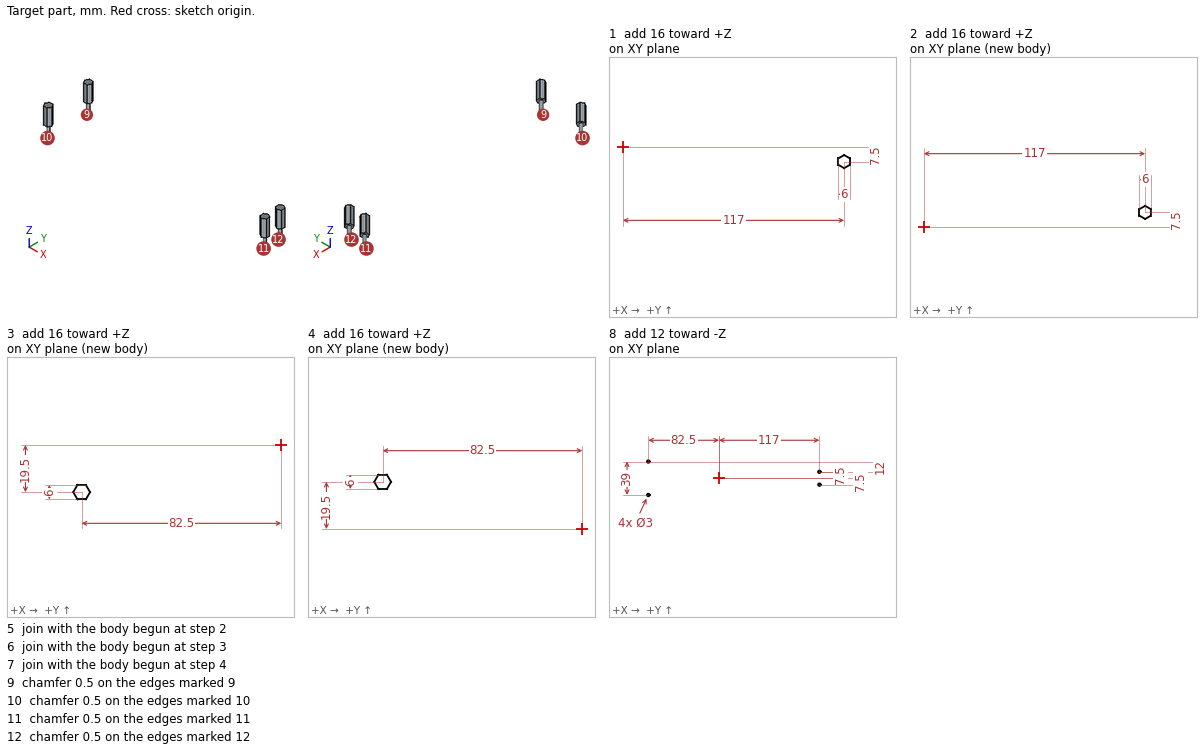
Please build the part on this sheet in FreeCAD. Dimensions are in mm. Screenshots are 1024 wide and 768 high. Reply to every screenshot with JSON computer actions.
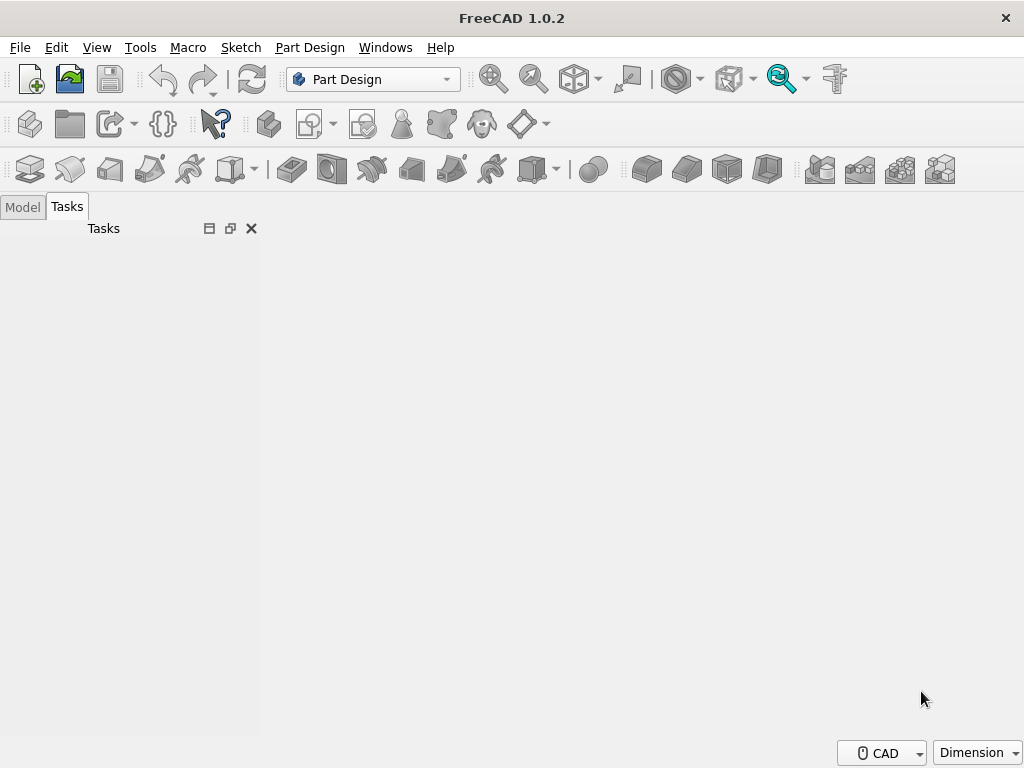
{"action": "left_click", "coordinate": [30, 80]}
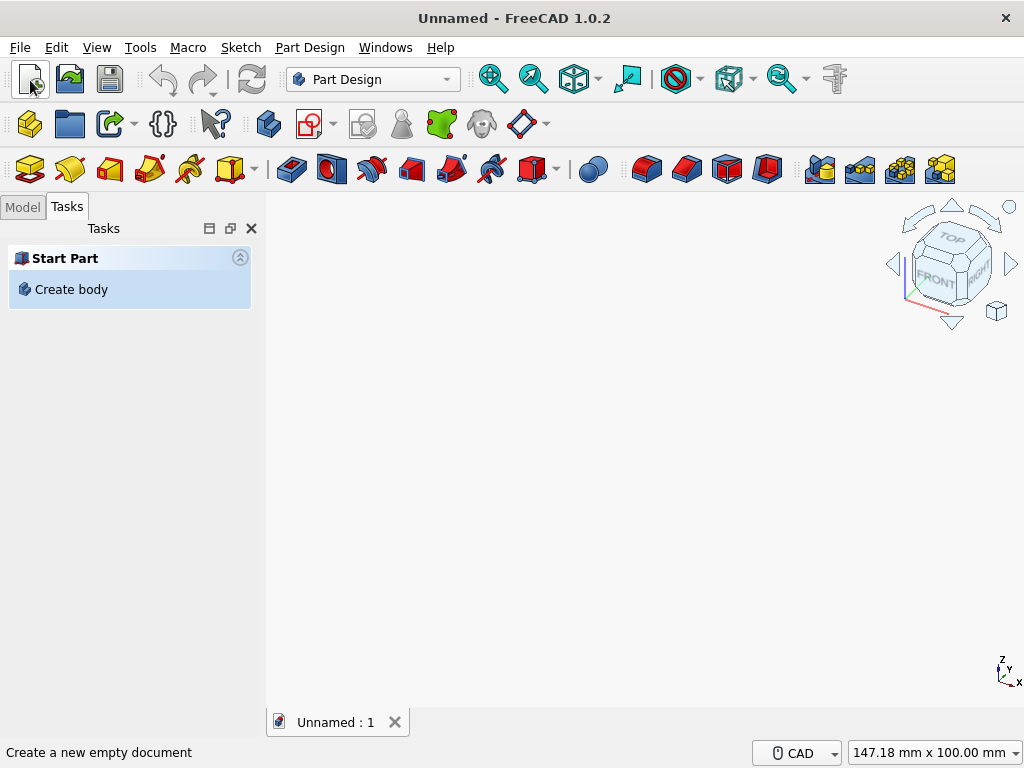
{"action": "left_click", "coordinate": [310, 124]}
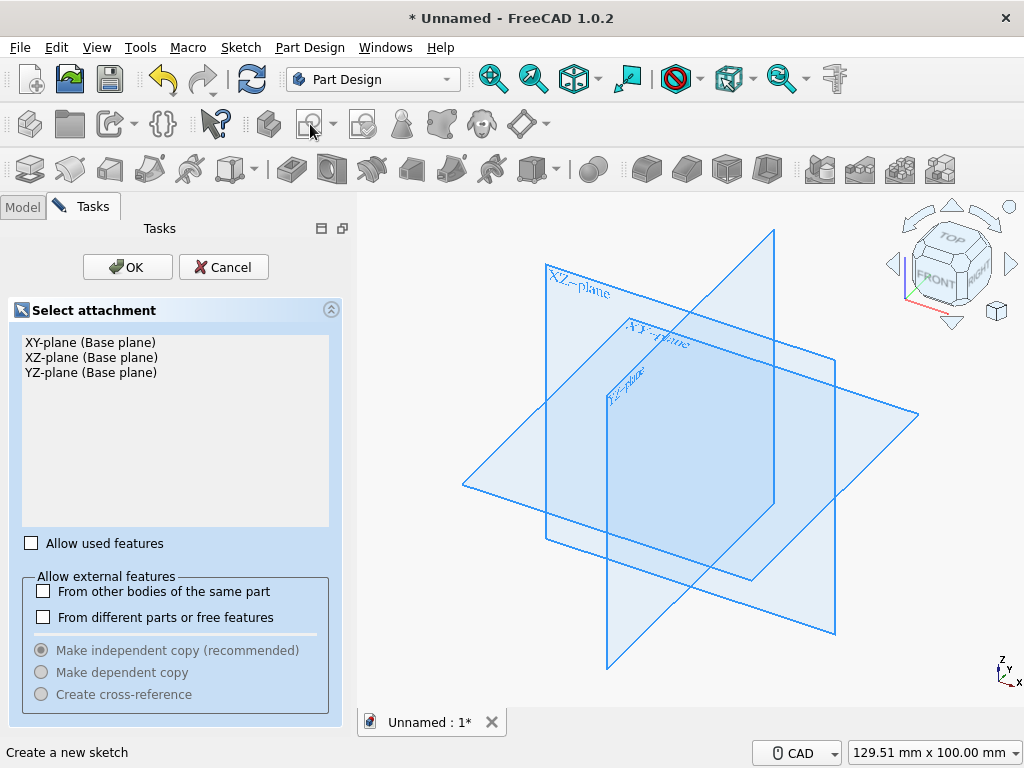
{"action": "left_click", "coordinate": [82, 342]}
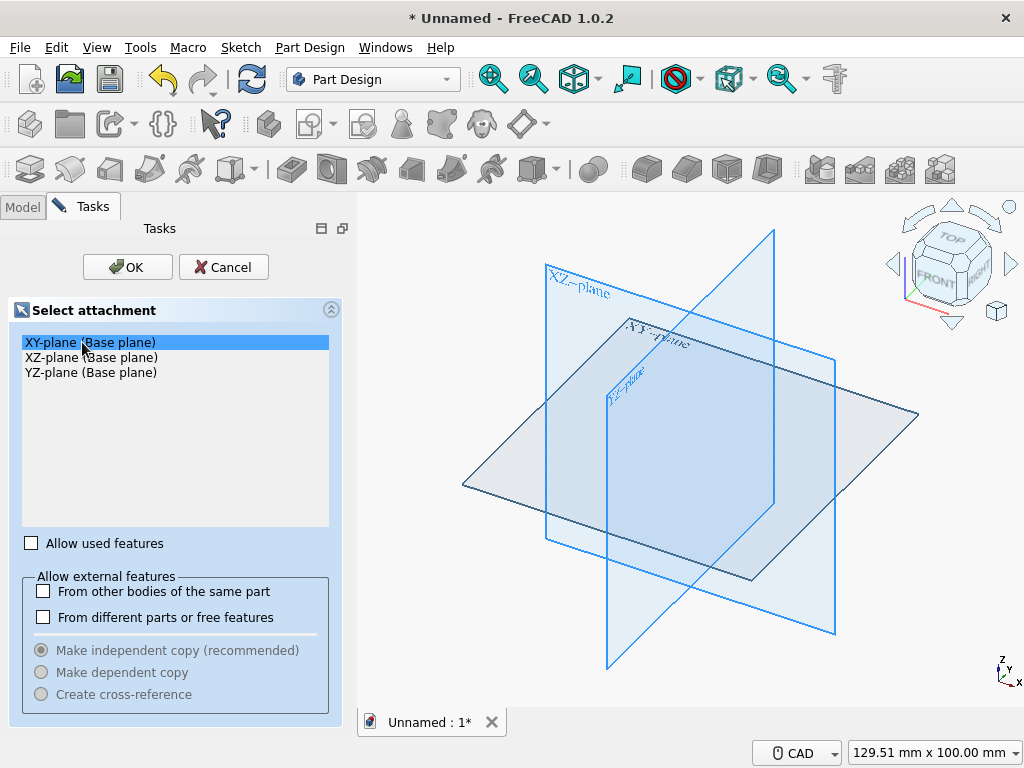
{"action": "left_click", "coordinate": [128, 267]}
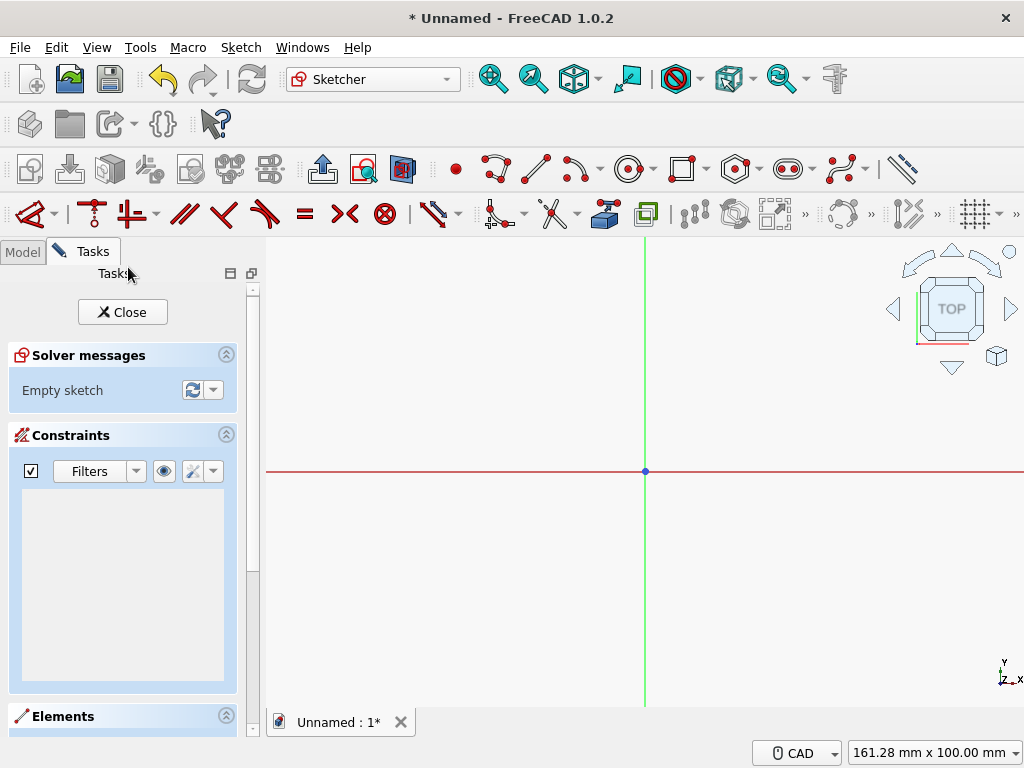
{"action": "scroll", "coordinate": [576, 472], "scroll_direction": "down", "scroll_amount": 5}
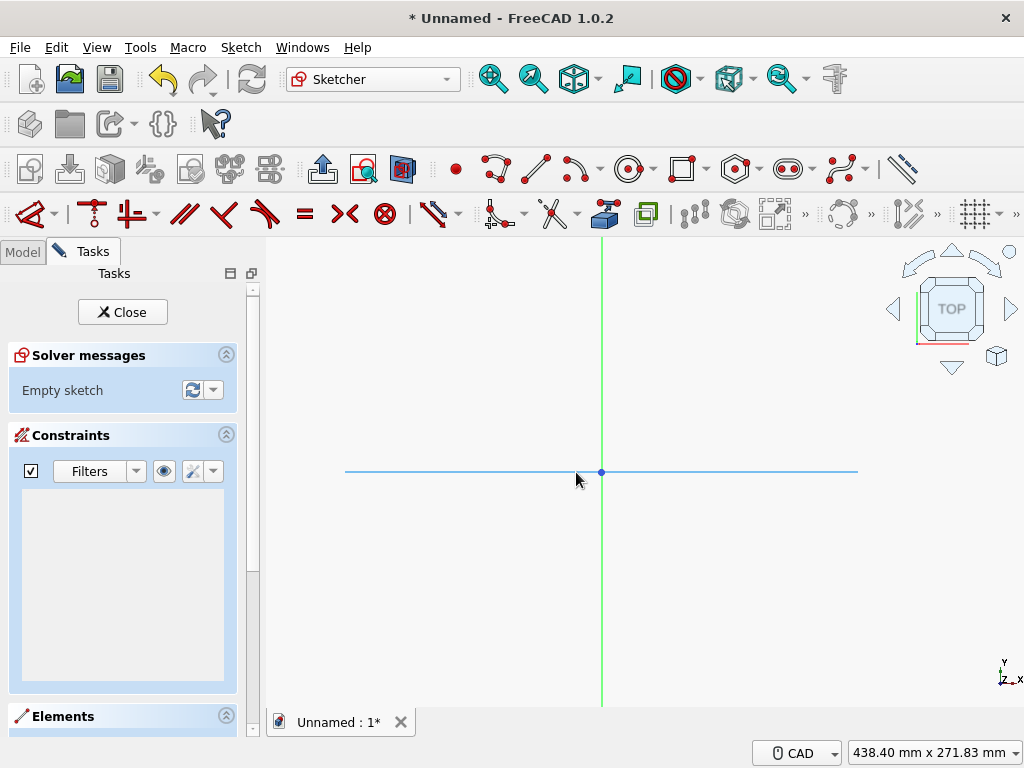
{"action": "scroll", "coordinate": [816, 486], "scroll_direction": "up", "scroll_amount": 15}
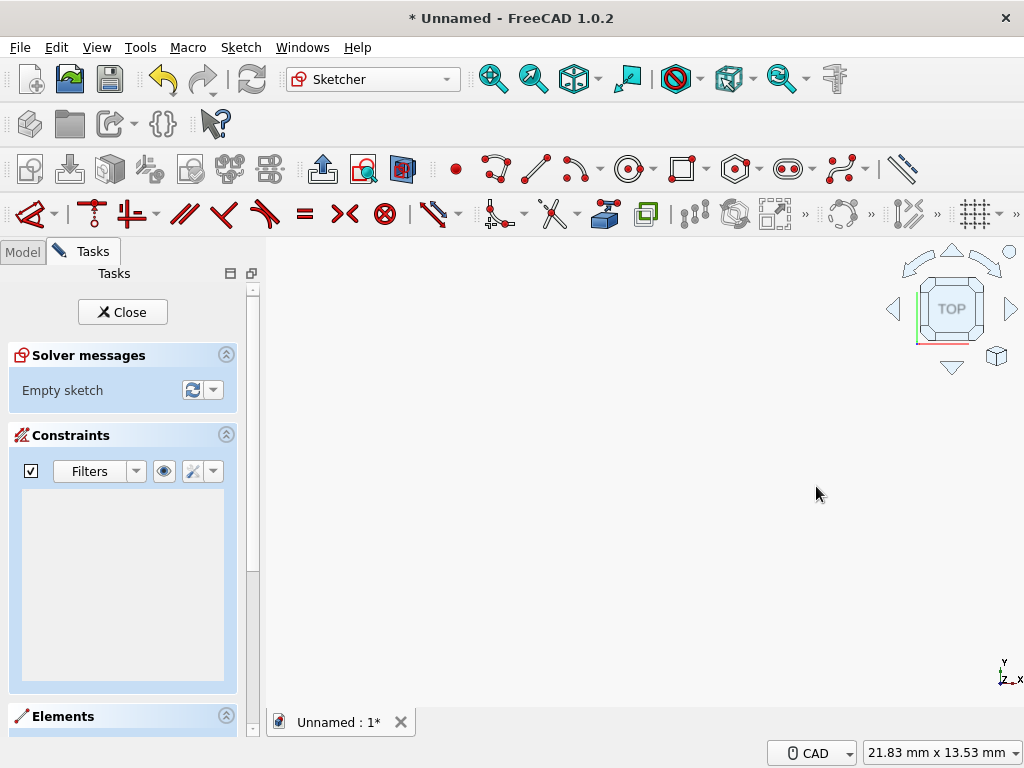
{"action": "left_click", "coordinate": [736, 170]}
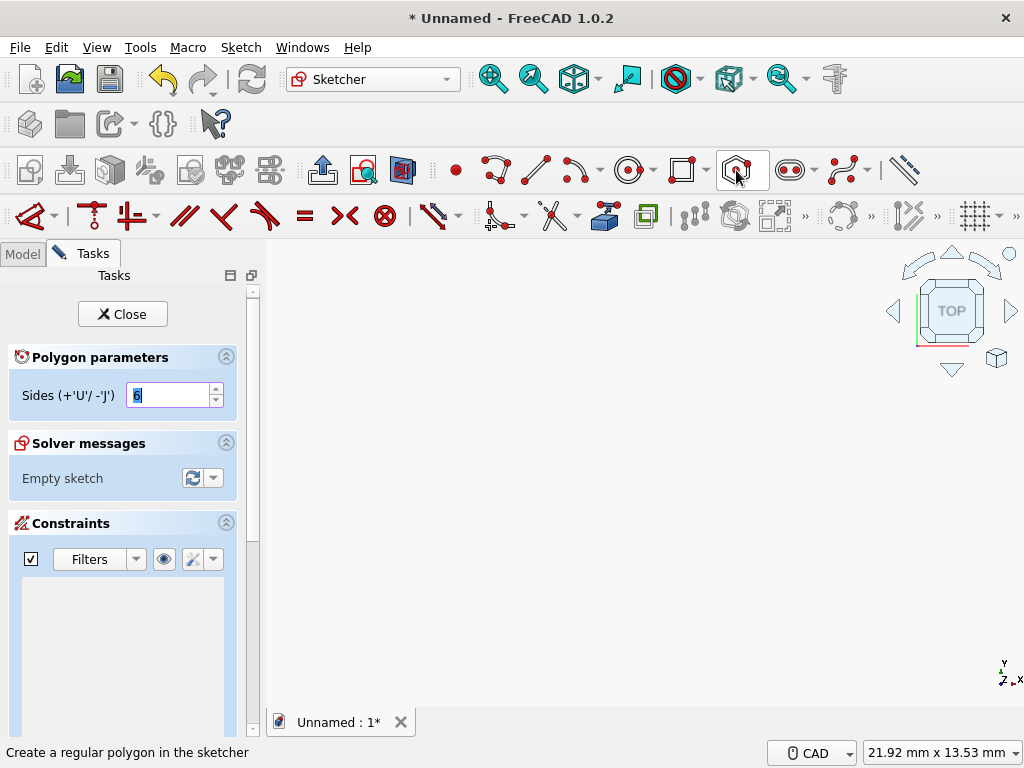
{"action": "left_click", "coordinate": [560, 463]}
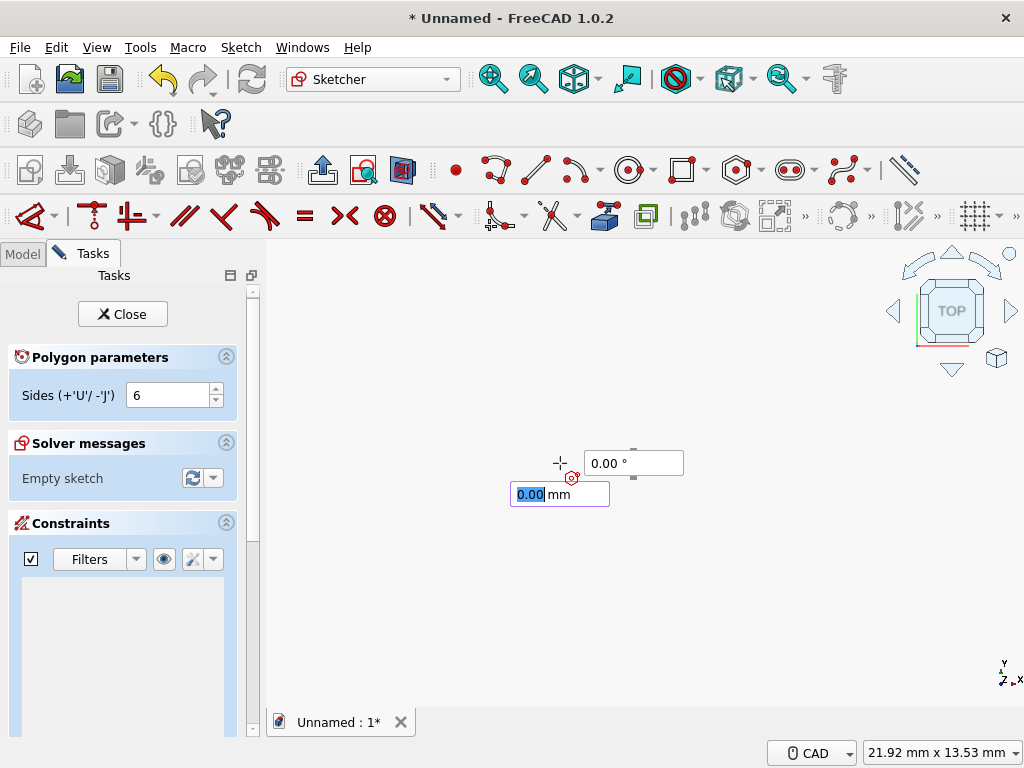
{"action": "left_click", "coordinate": [560, 582]}
{"action": "right_click", "coordinate": [560, 582]}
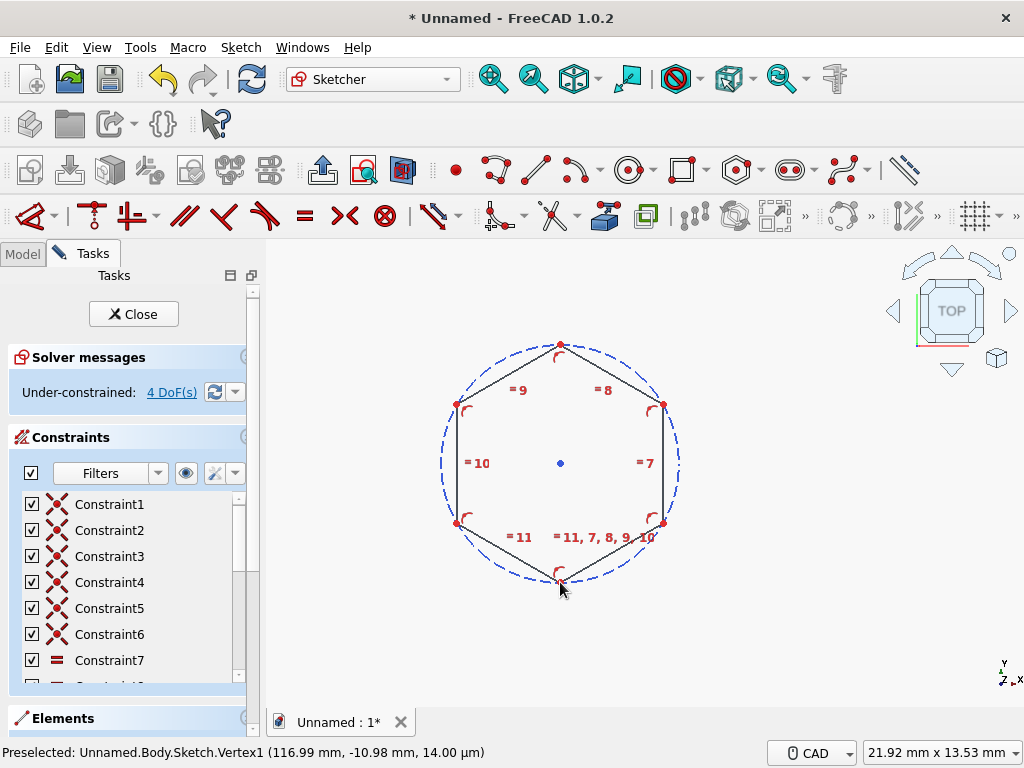
{"action": "left_click", "coordinate": [663, 488]}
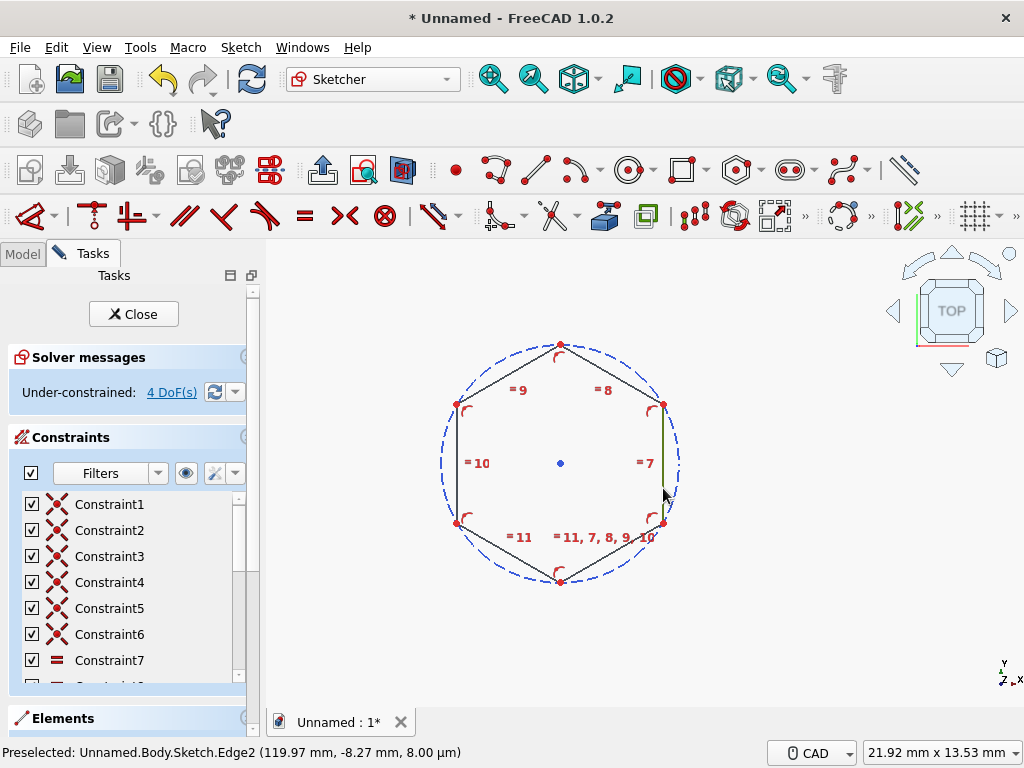
{"action": "left_click", "coordinate": [158, 216]}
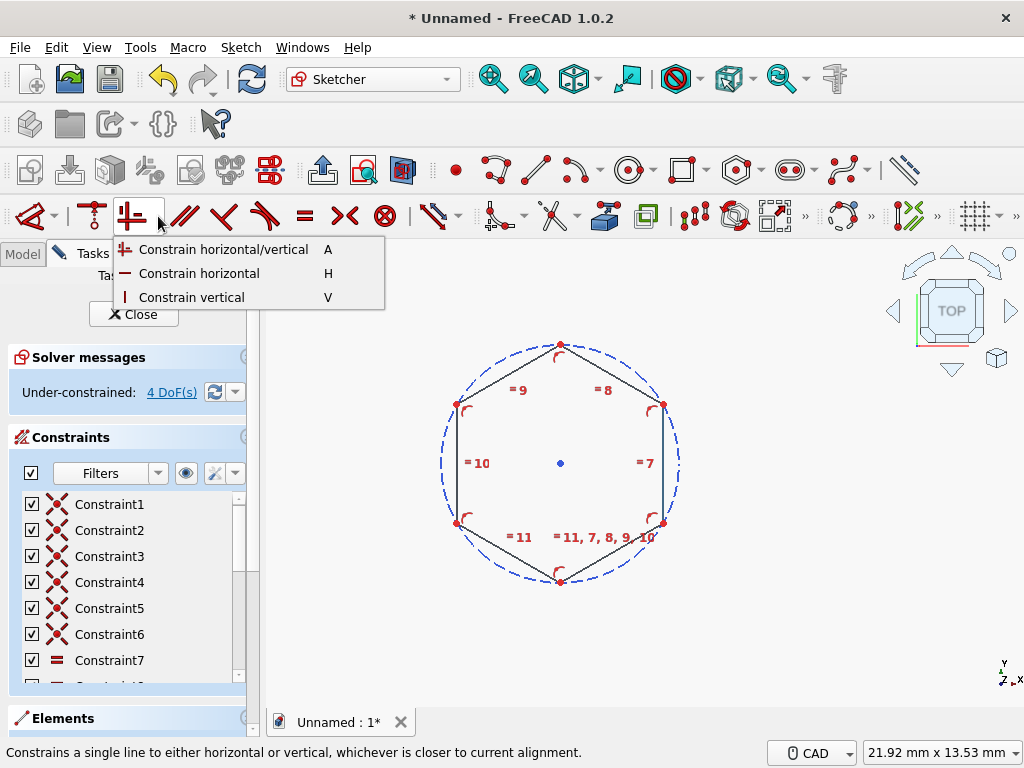
{"action": "left_click", "coordinate": [249, 297]}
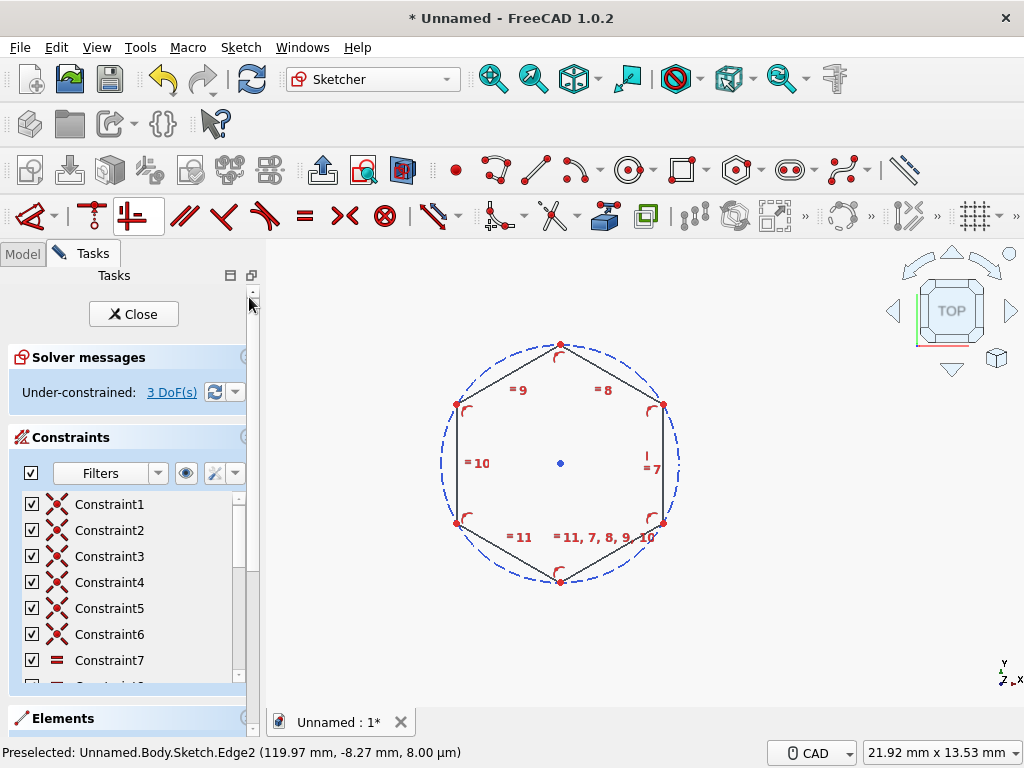
{"action": "left_click", "coordinate": [30, 216]}